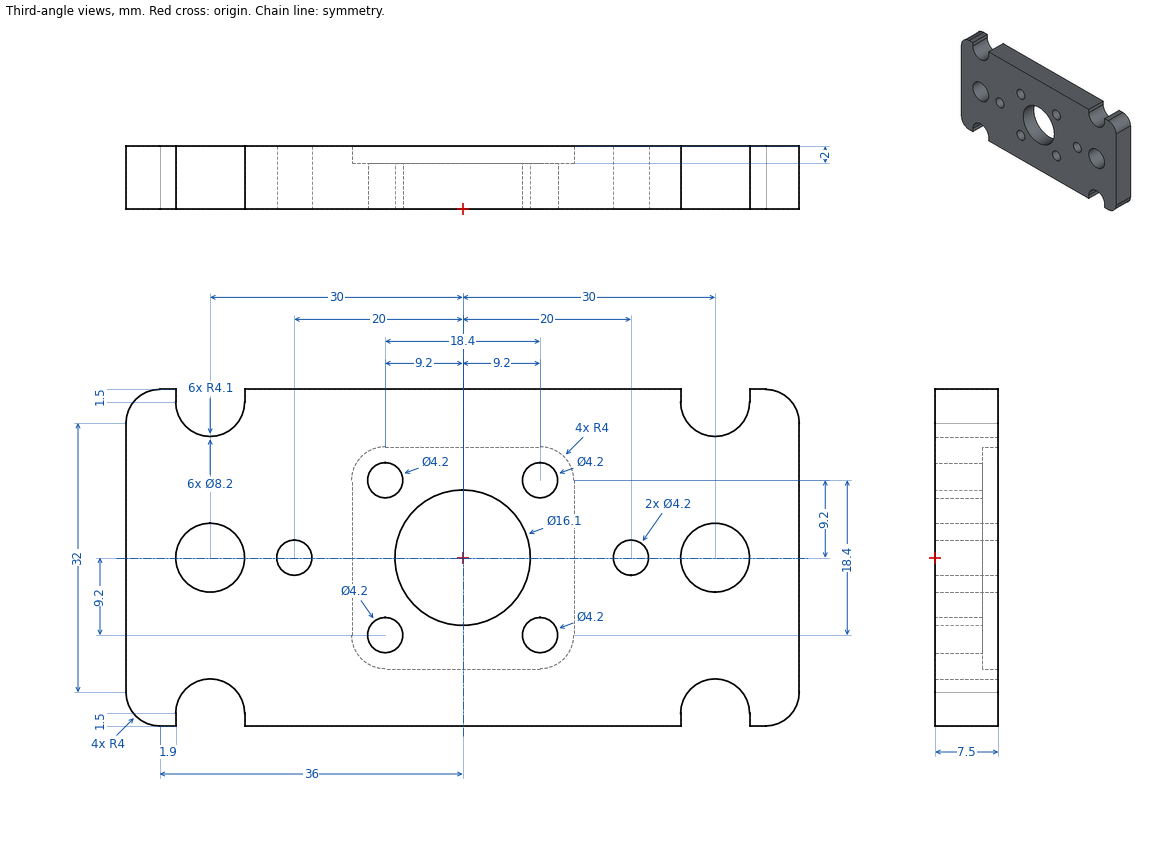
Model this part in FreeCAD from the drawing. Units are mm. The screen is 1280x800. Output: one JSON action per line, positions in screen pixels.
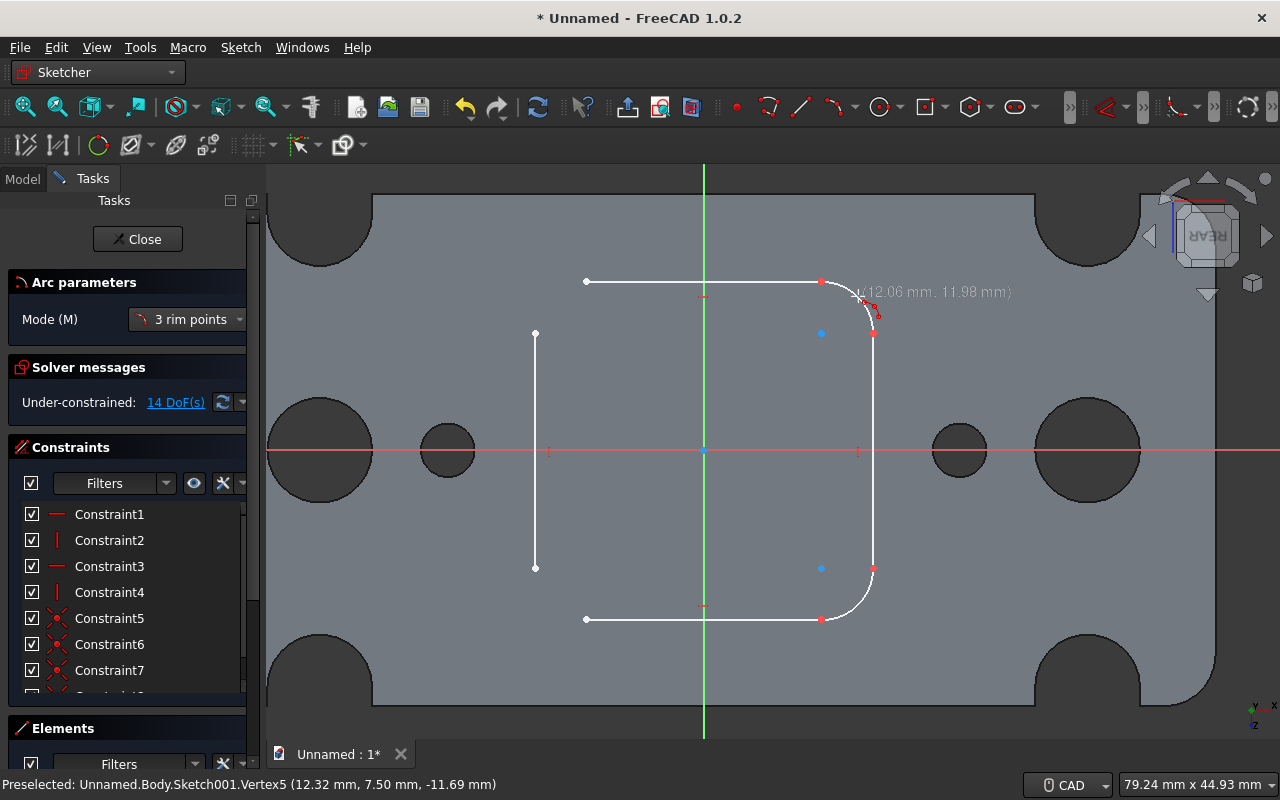
{"action": "left_click", "coordinate": [586, 282]}
{"action": "left_click", "coordinate": [535, 334]}
{"action": "left_click", "coordinate": [550, 296]}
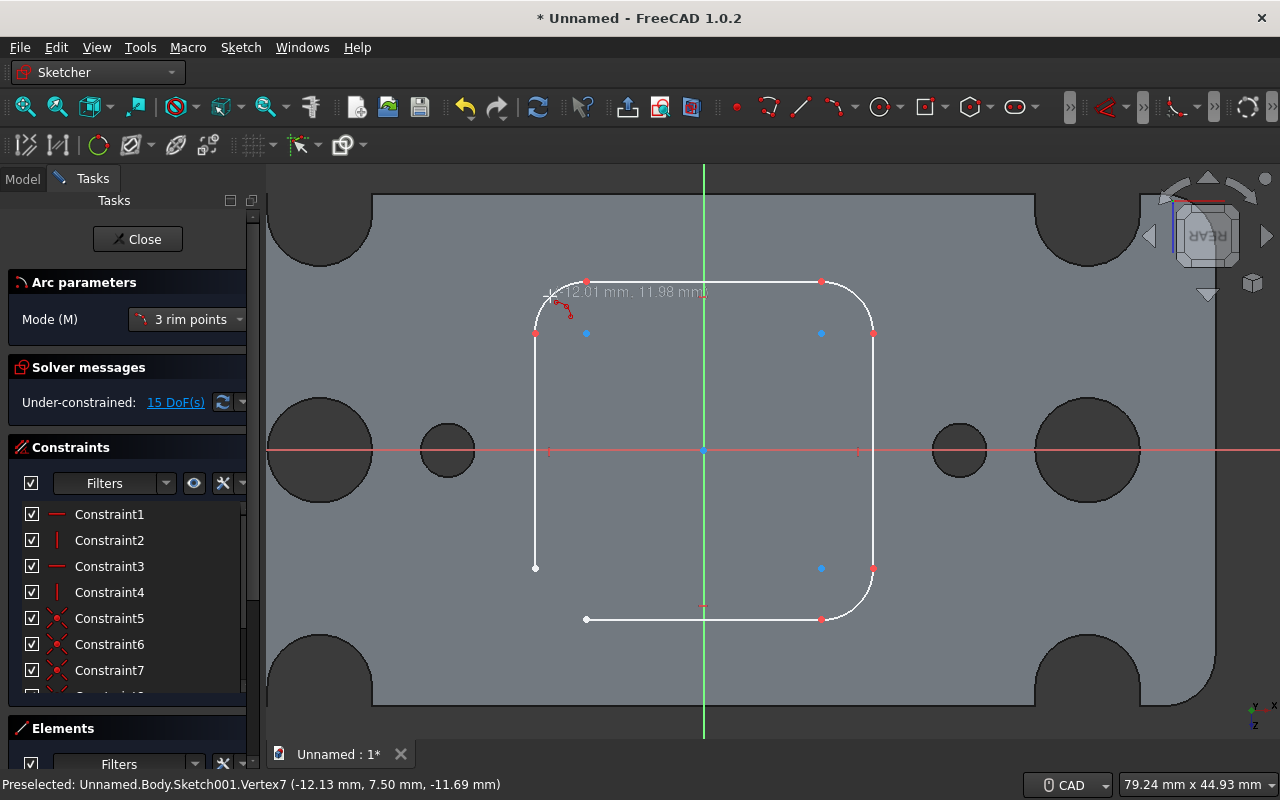
{"action": "left_click", "coordinate": [535, 569]}
{"action": "left_click", "coordinate": [586, 620]}
{"action": "left_click", "coordinate": [550, 604]}
{"action": "key", "text": "Escape"}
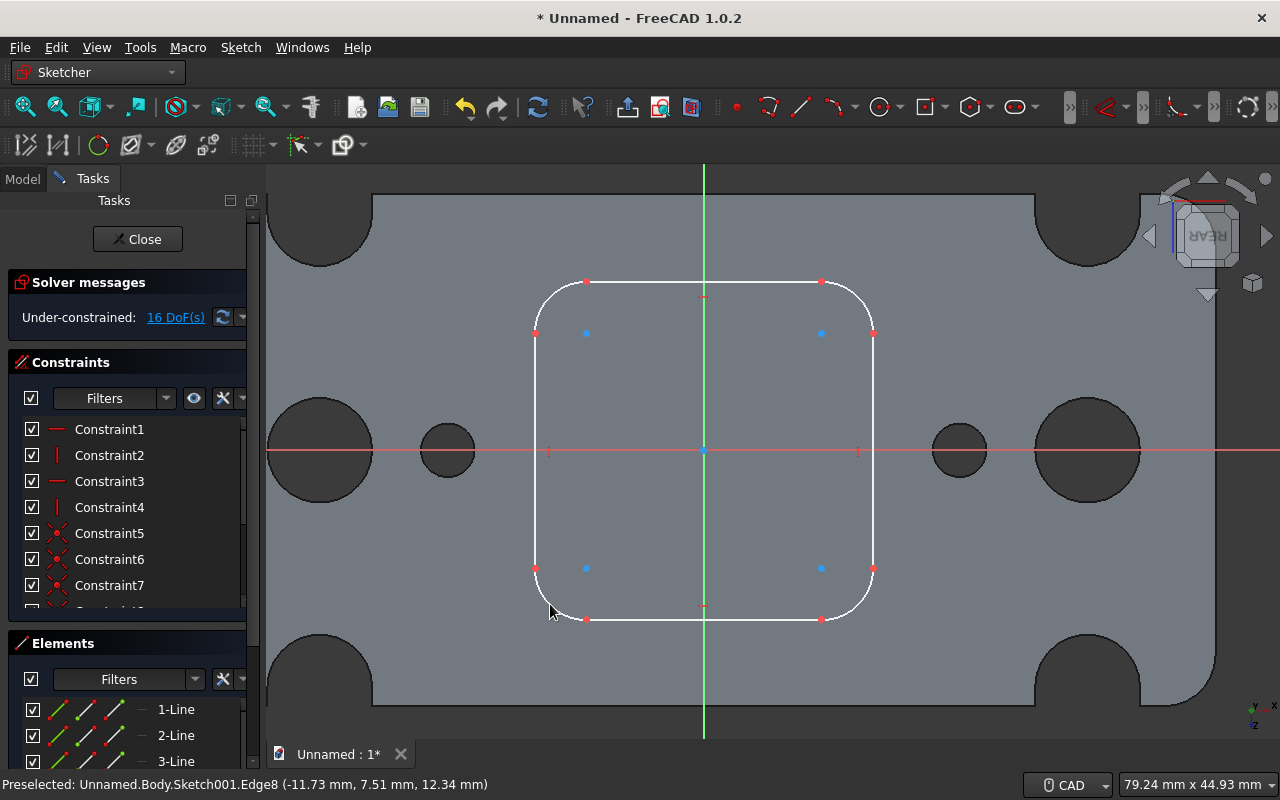
{"action": "left_click", "coordinate": [657, 620]}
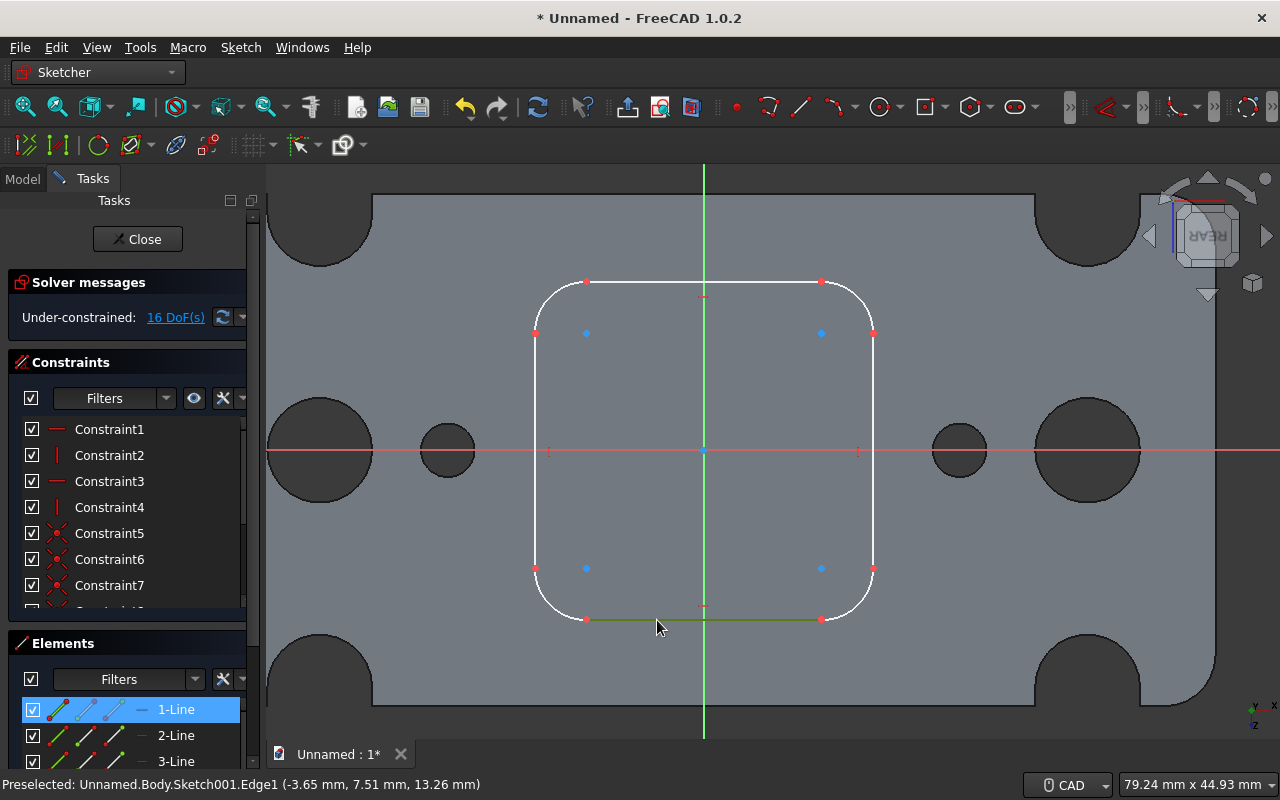
{"action": "left_click", "coordinate": [844, 615]}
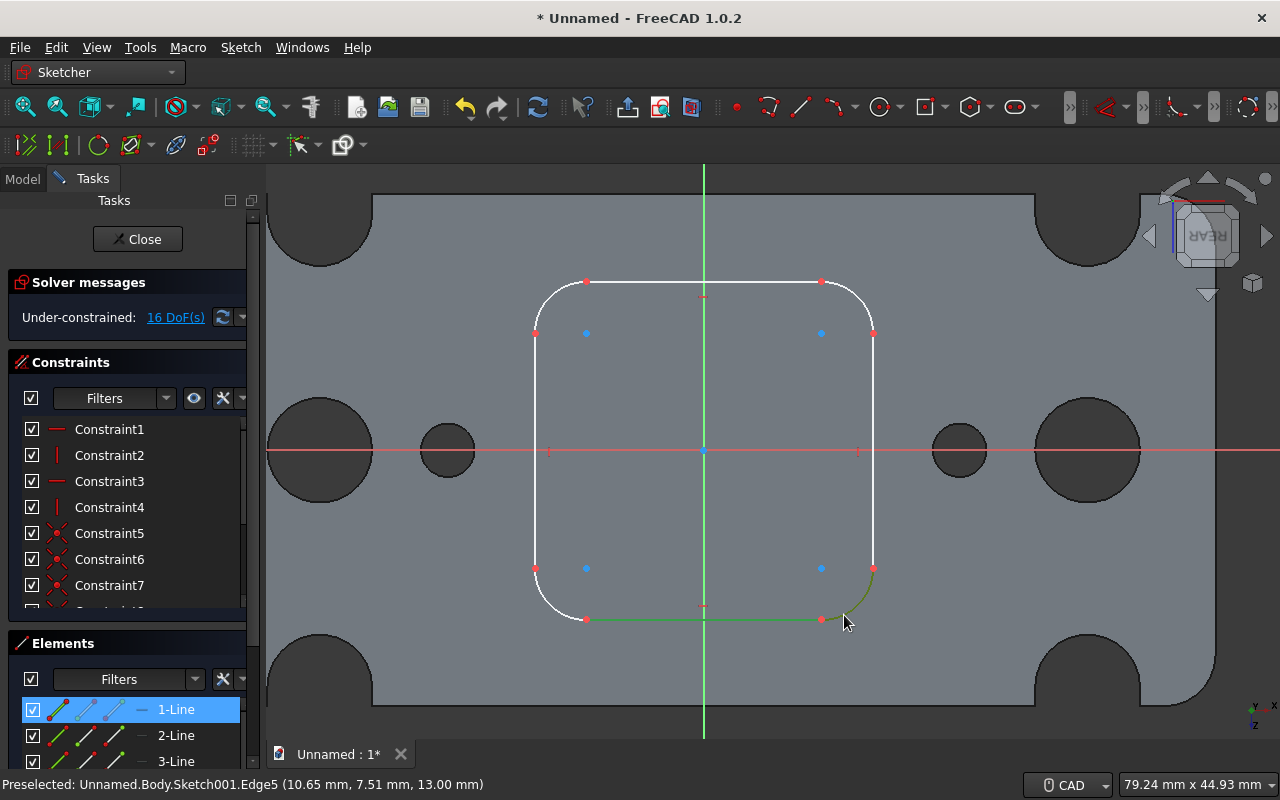
{"action": "key", "text": "t"}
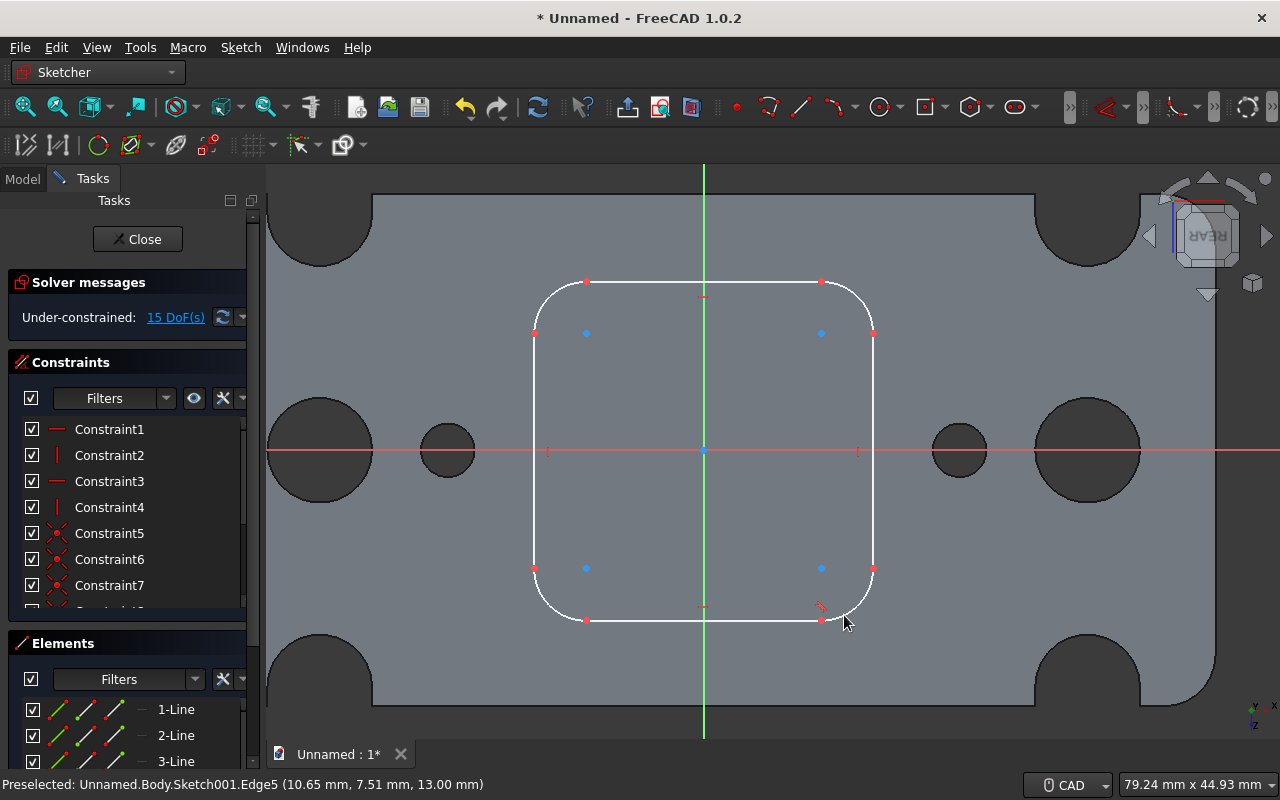
{"action": "left_click", "coordinate": [657, 621]}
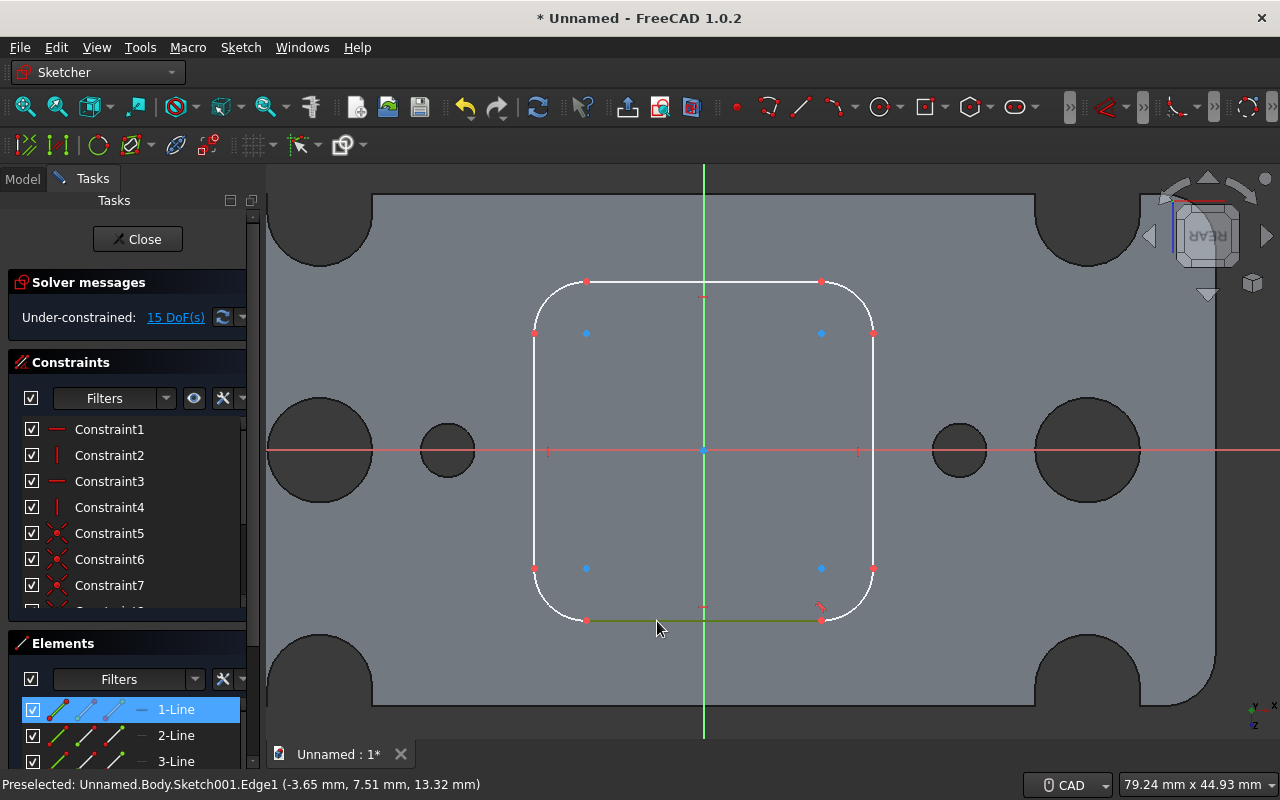
{"action": "left_click", "coordinate": [540, 592]}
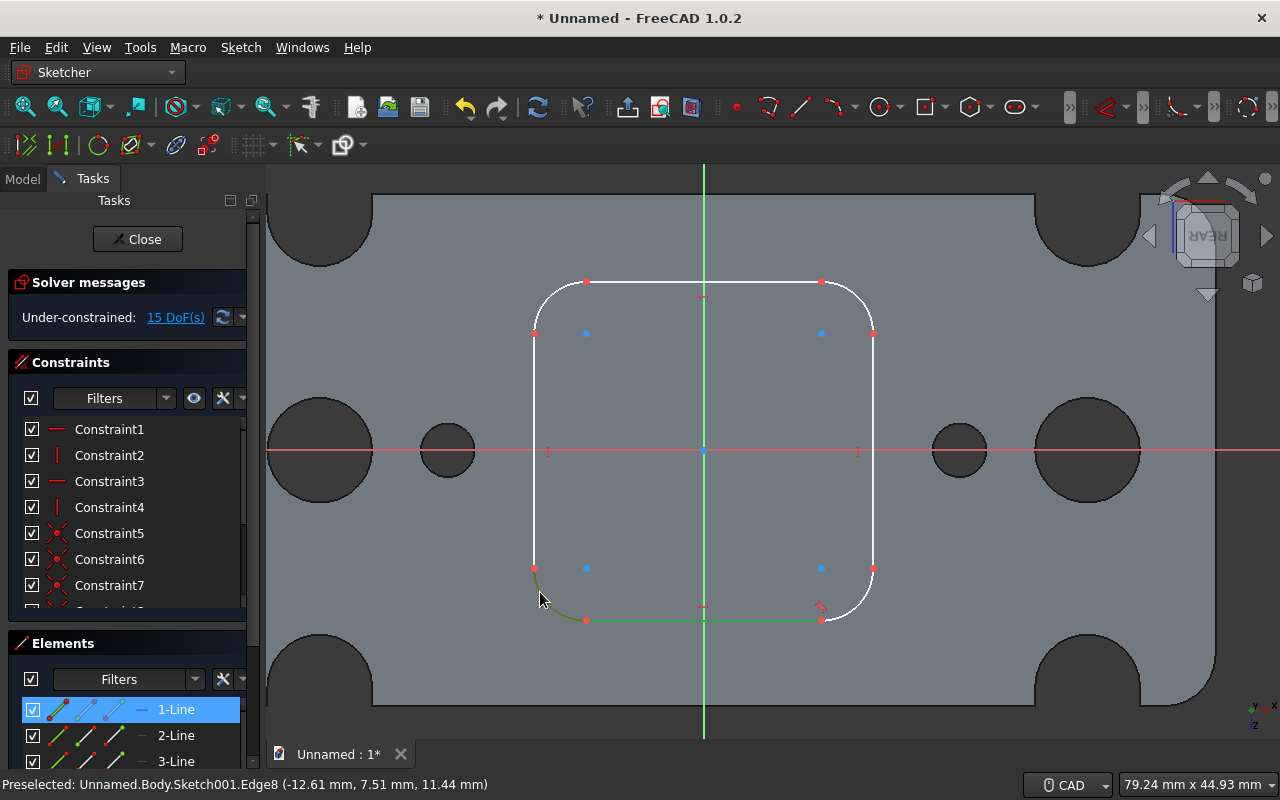
{"action": "key", "text": "t"}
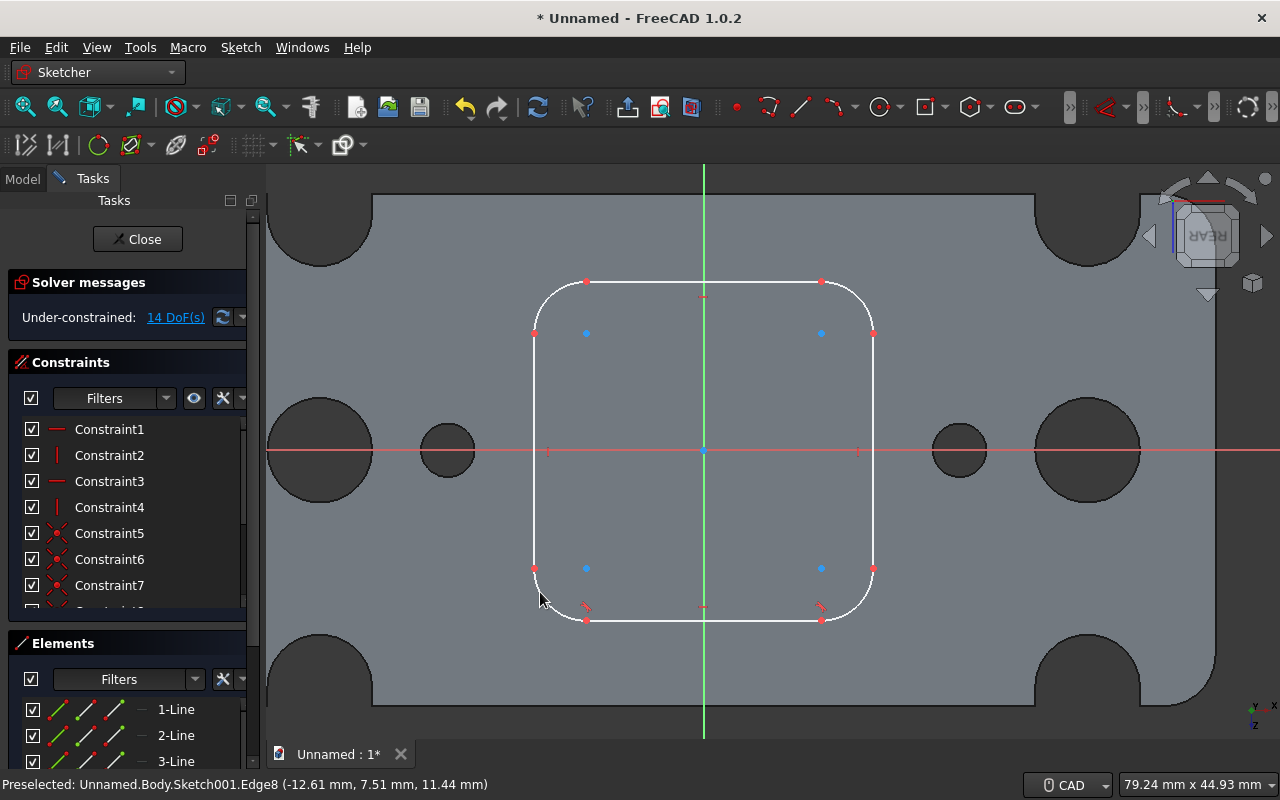
{"action": "left_click", "coordinate": [873, 498]}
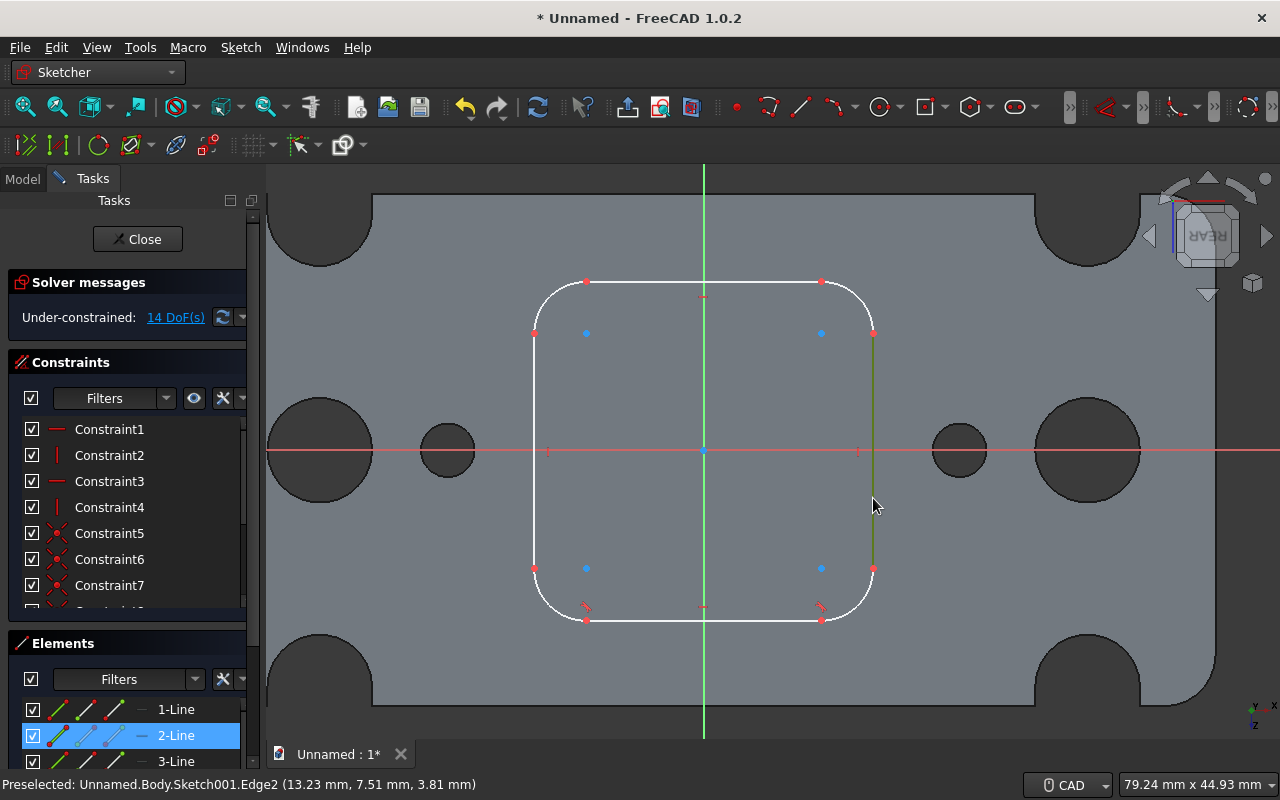
{"action": "left_click", "coordinate": [845, 615]}